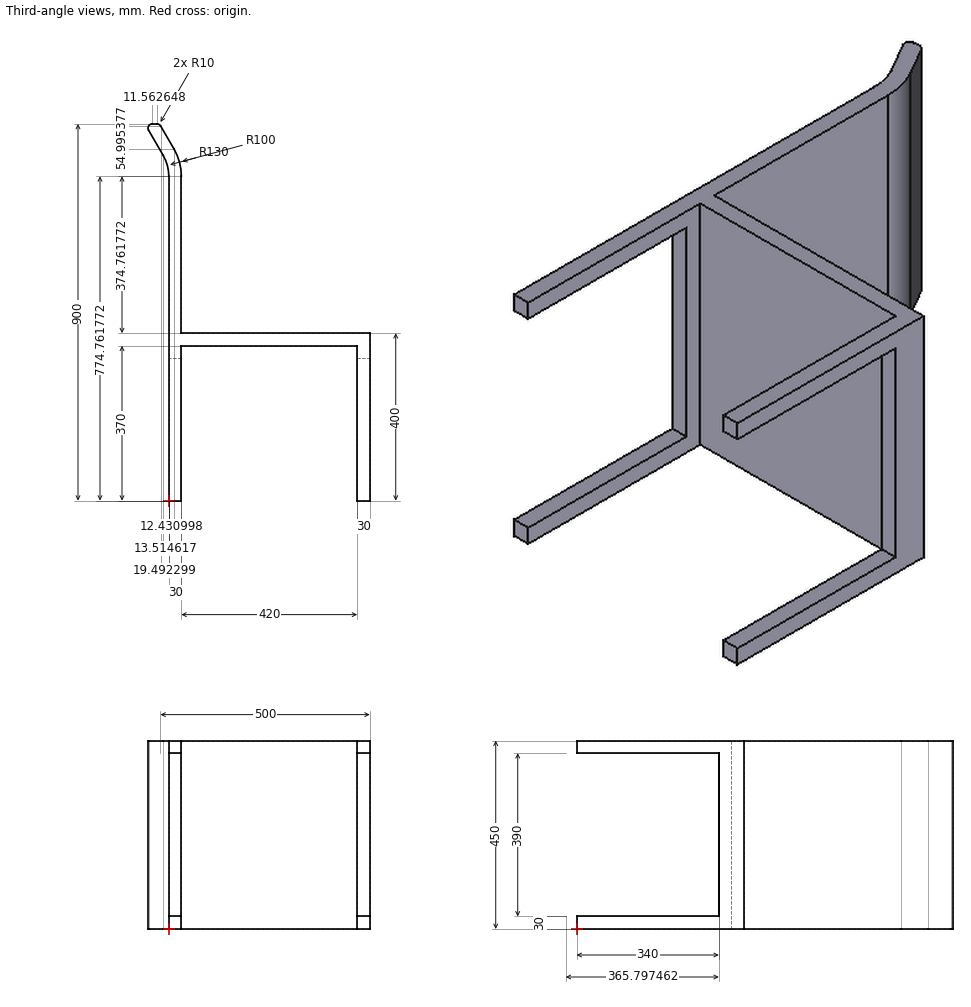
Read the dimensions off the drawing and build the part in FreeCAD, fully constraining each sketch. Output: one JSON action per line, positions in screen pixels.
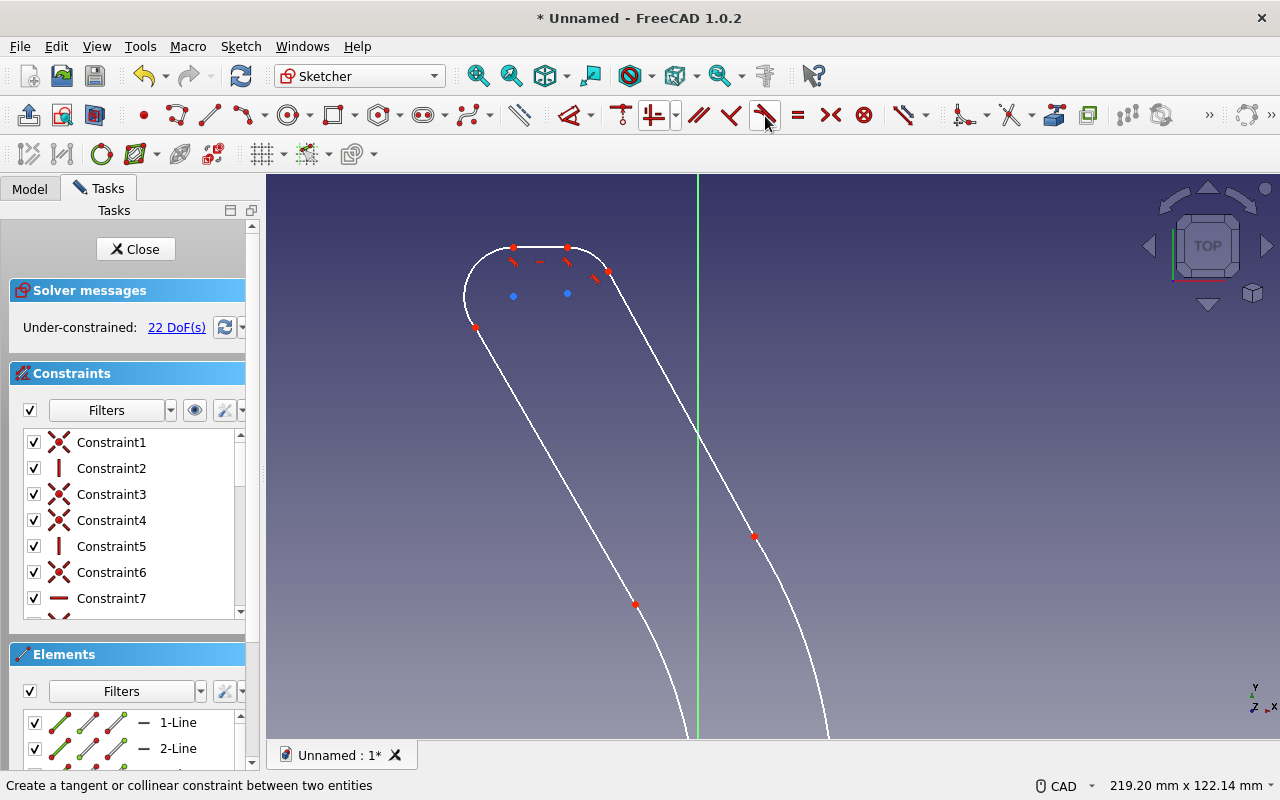
{"action": "scroll", "coordinate": [606, 269], "scroll_direction": "down", "scroll_amount": 12}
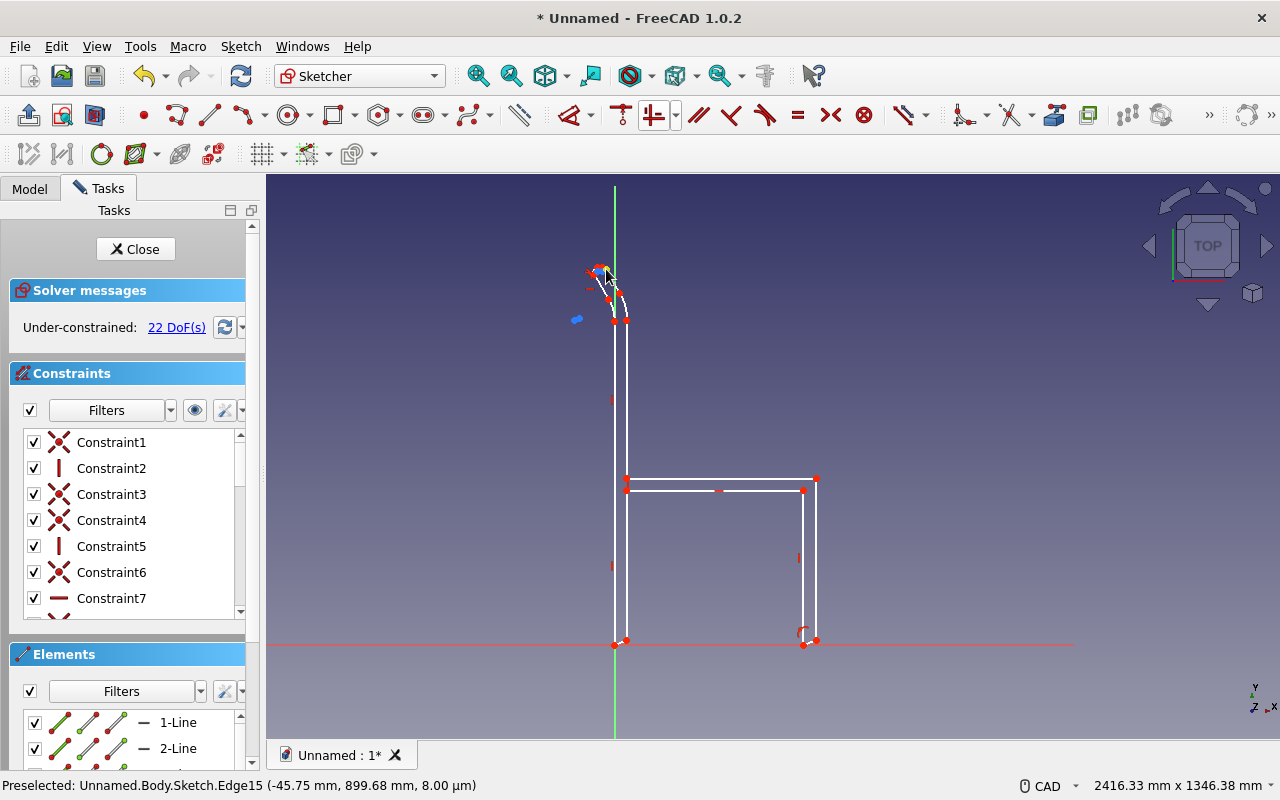
{"action": "scroll", "coordinate": [599, 282], "scroll_direction": "up", "scroll_amount": 3}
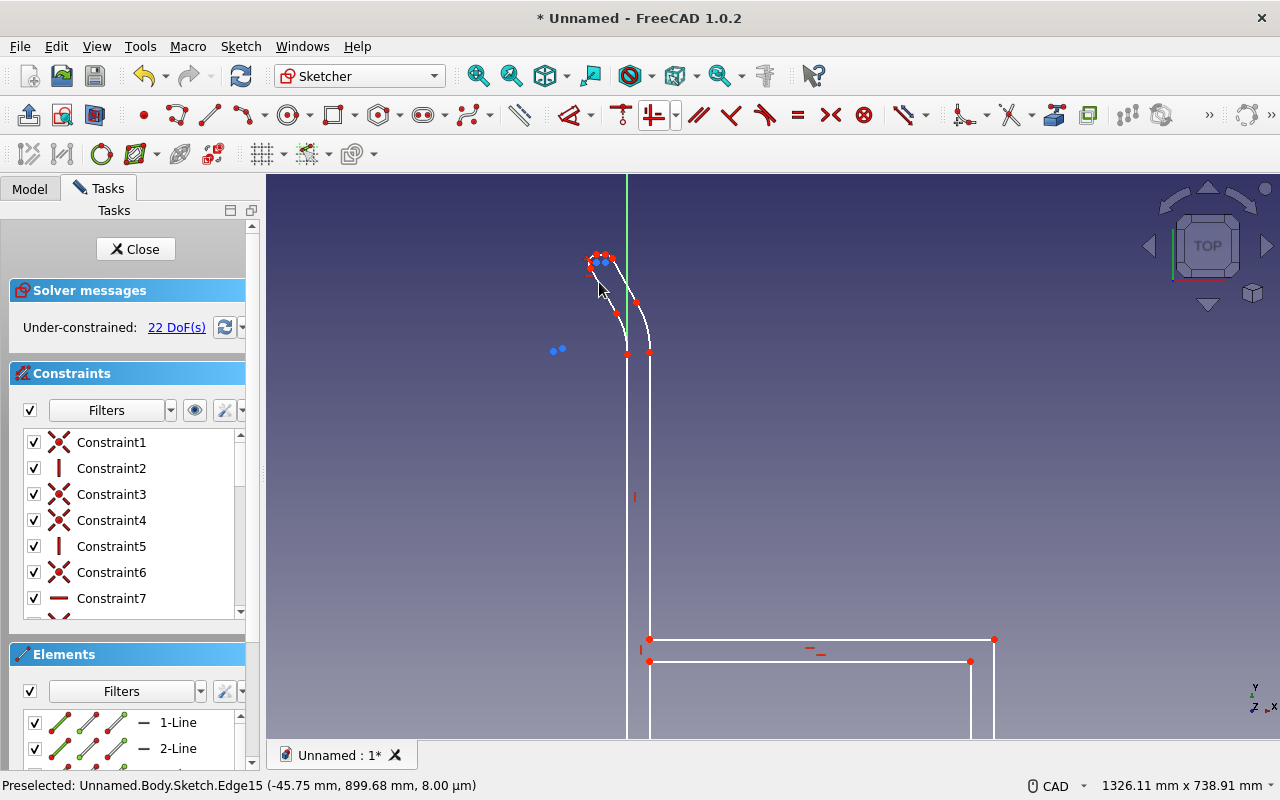
{"action": "left_click", "coordinate": [598, 282]}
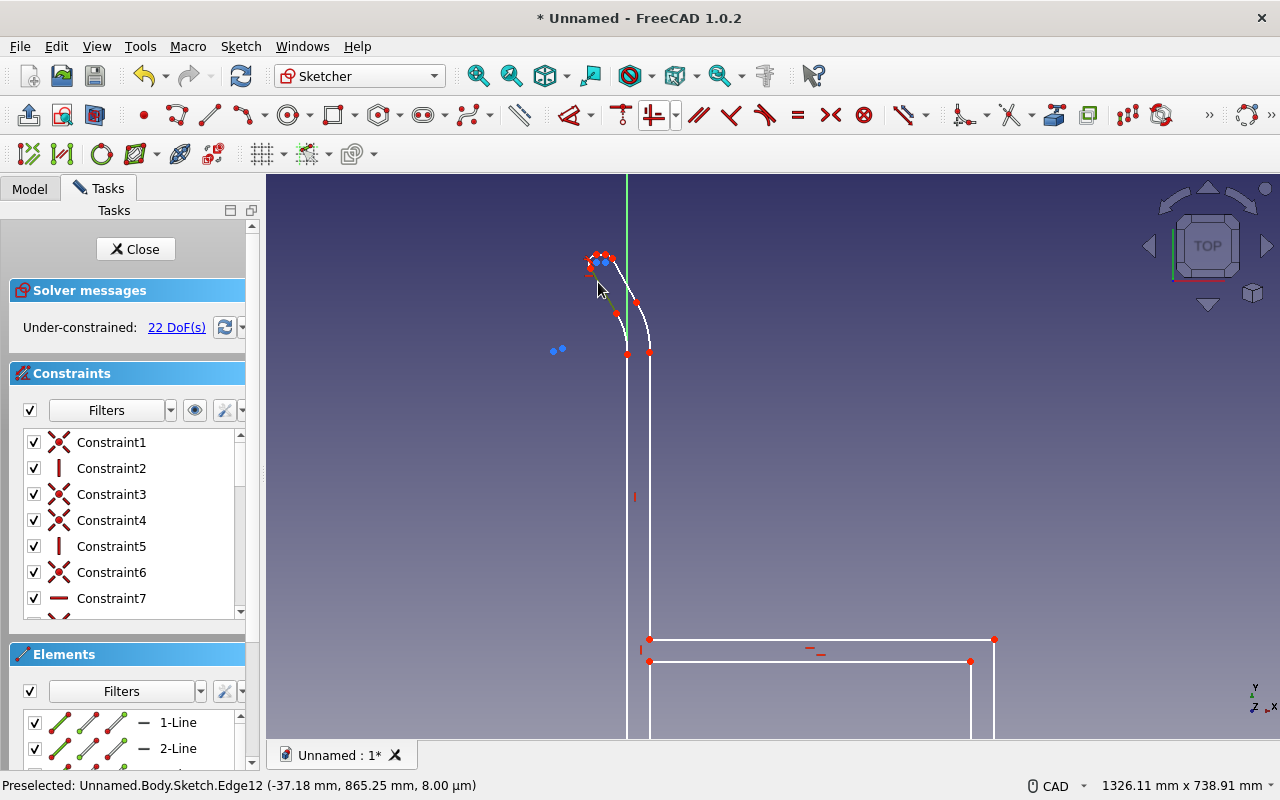
{"action": "scroll", "coordinate": [589, 259], "scroll_direction": "up", "scroll_amount": 3}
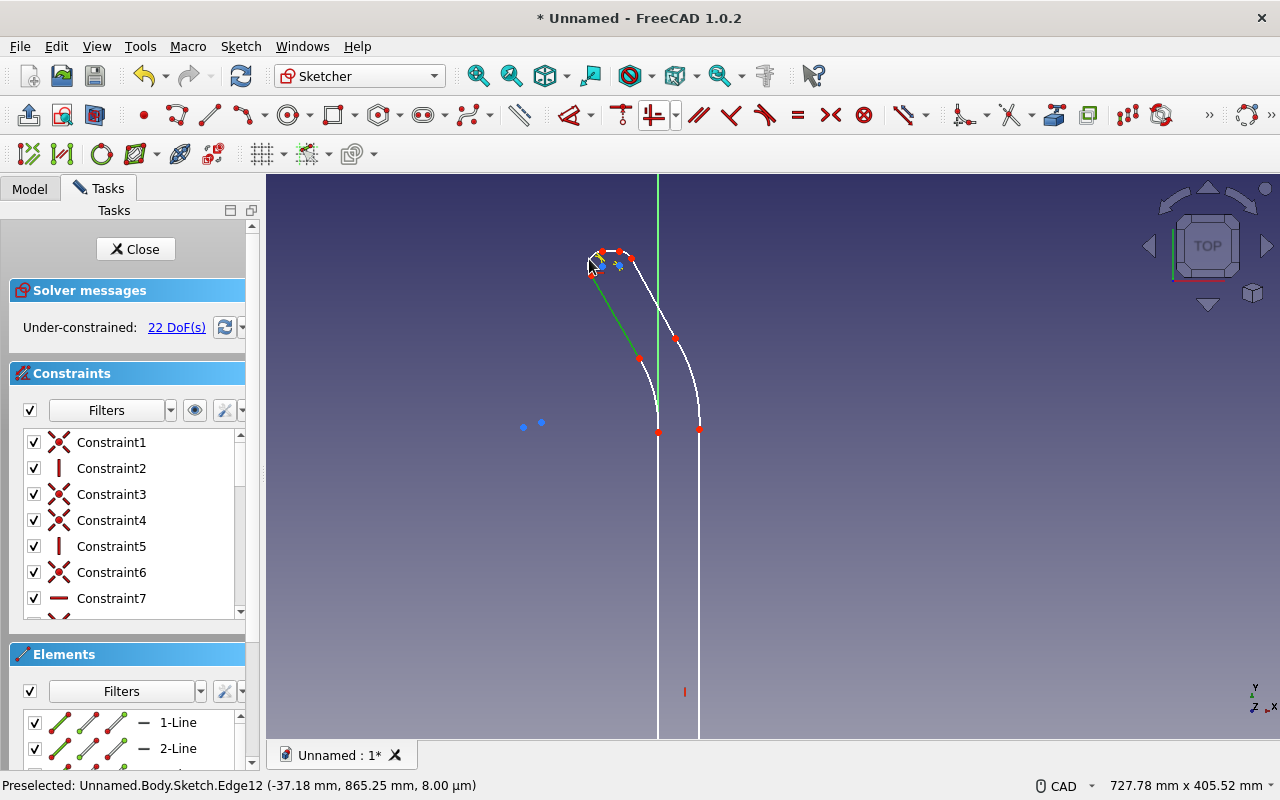
{"action": "left_click", "coordinate": [589, 260]}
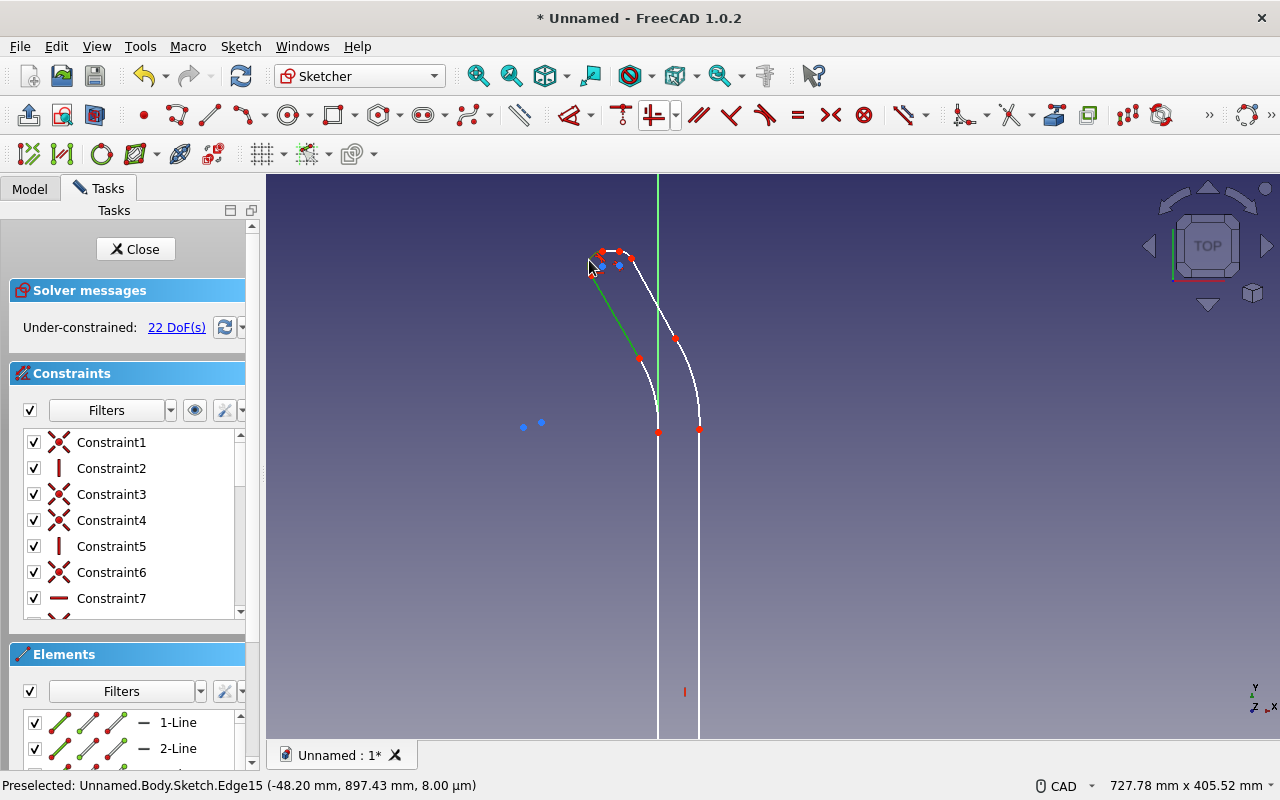
{"action": "left_click", "coordinate": [765, 116]}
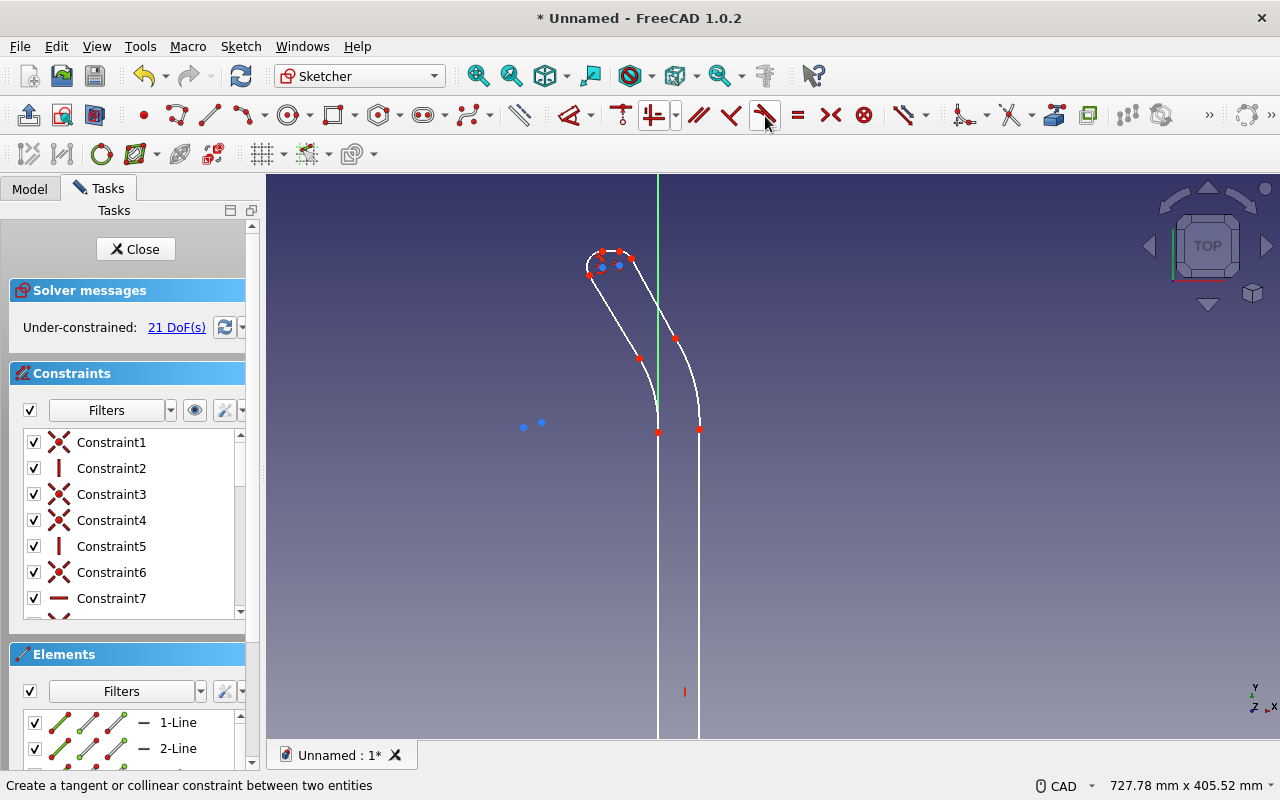
{"action": "scroll", "coordinate": [595, 274], "scroll_direction": "down", "scroll_amount": 6}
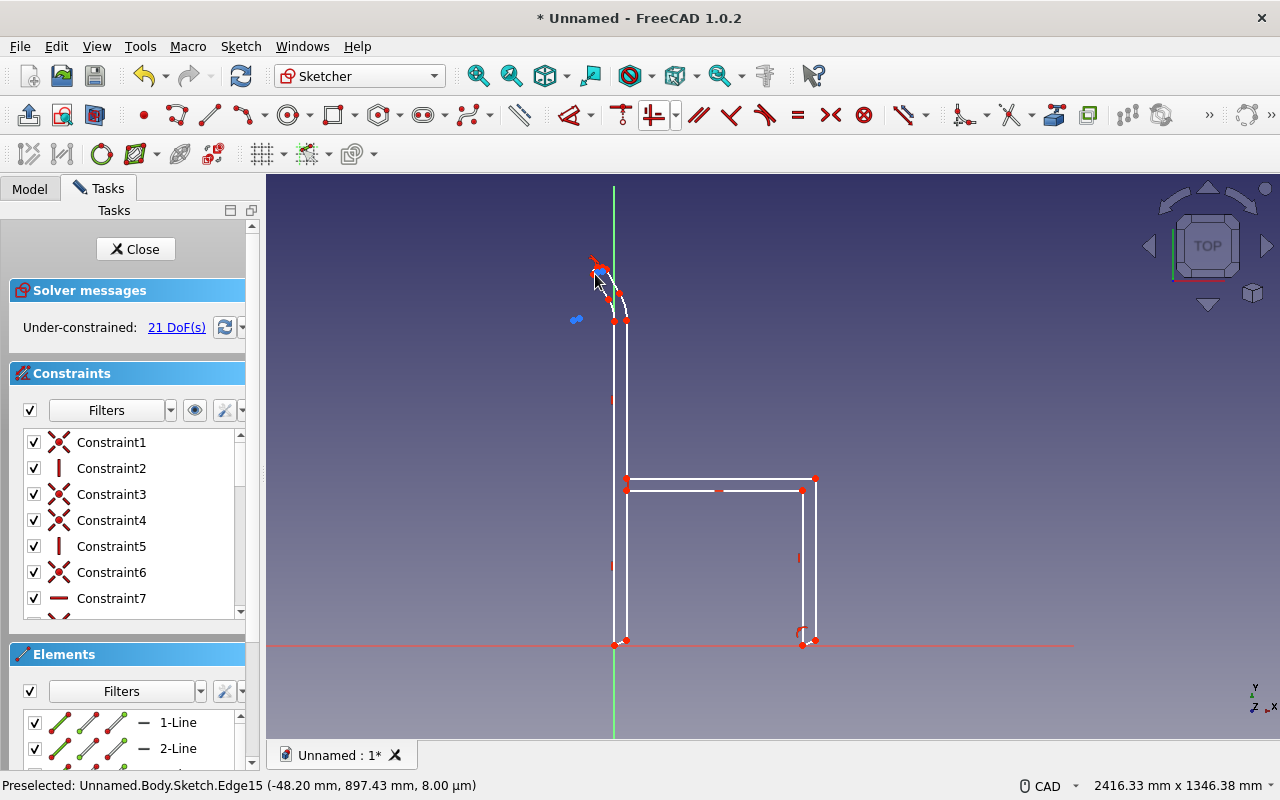
{"action": "scroll", "coordinate": [623, 642], "scroll_direction": "up", "scroll_amount": 7}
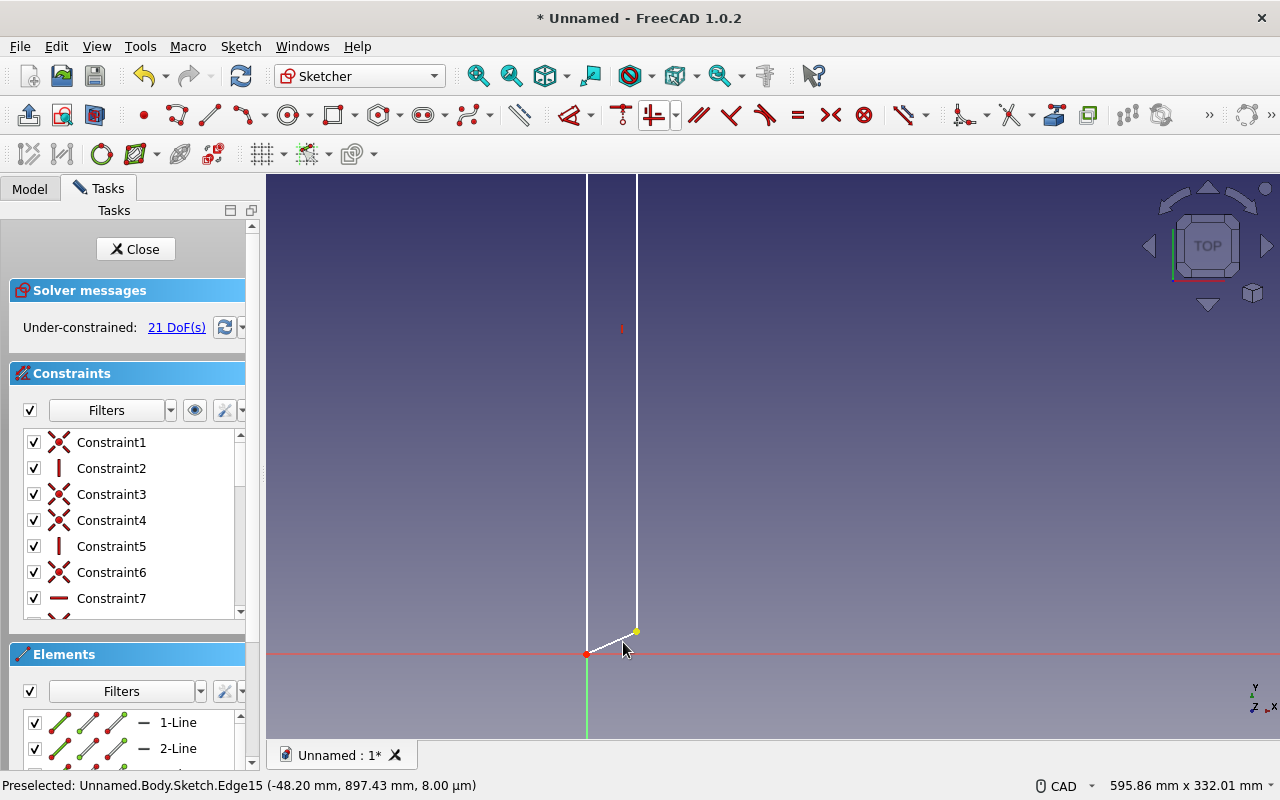
{"action": "left_click", "coordinate": [622, 639]}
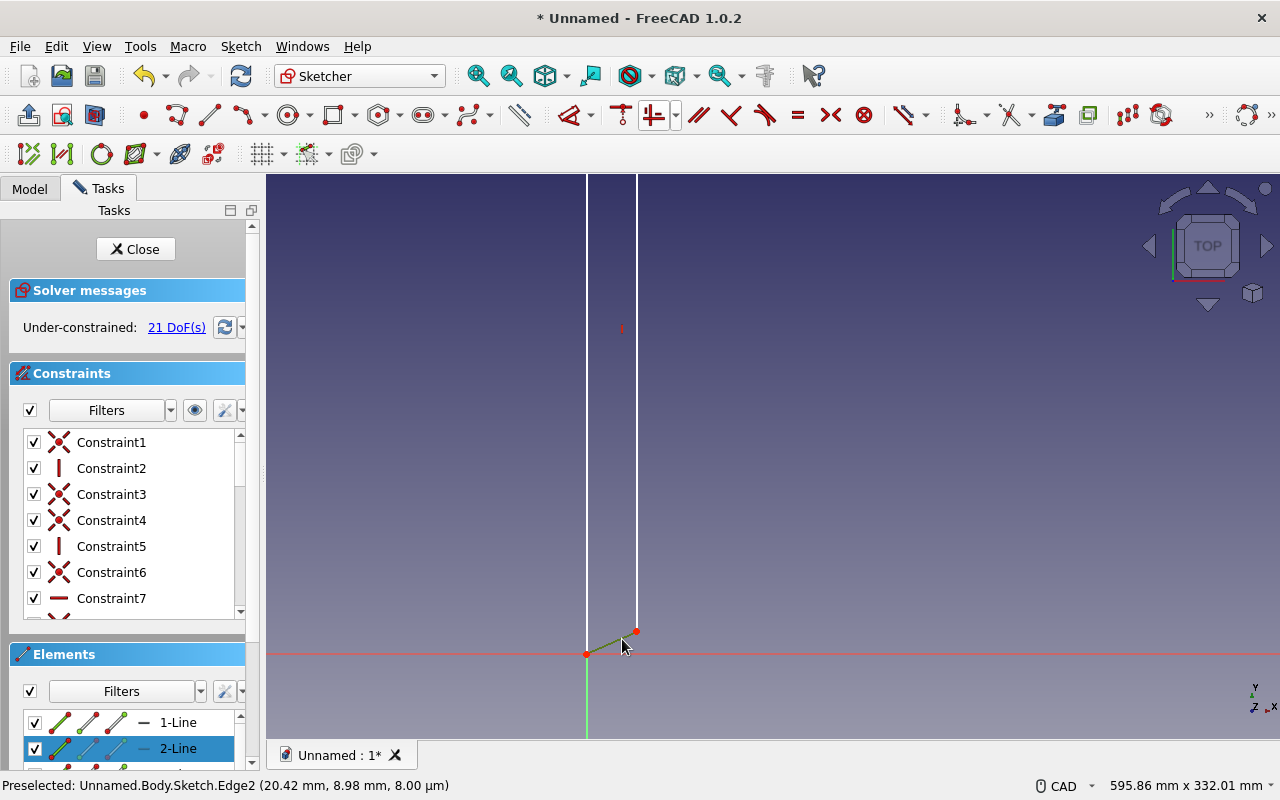
{"action": "left_click", "coordinate": [676, 116]}